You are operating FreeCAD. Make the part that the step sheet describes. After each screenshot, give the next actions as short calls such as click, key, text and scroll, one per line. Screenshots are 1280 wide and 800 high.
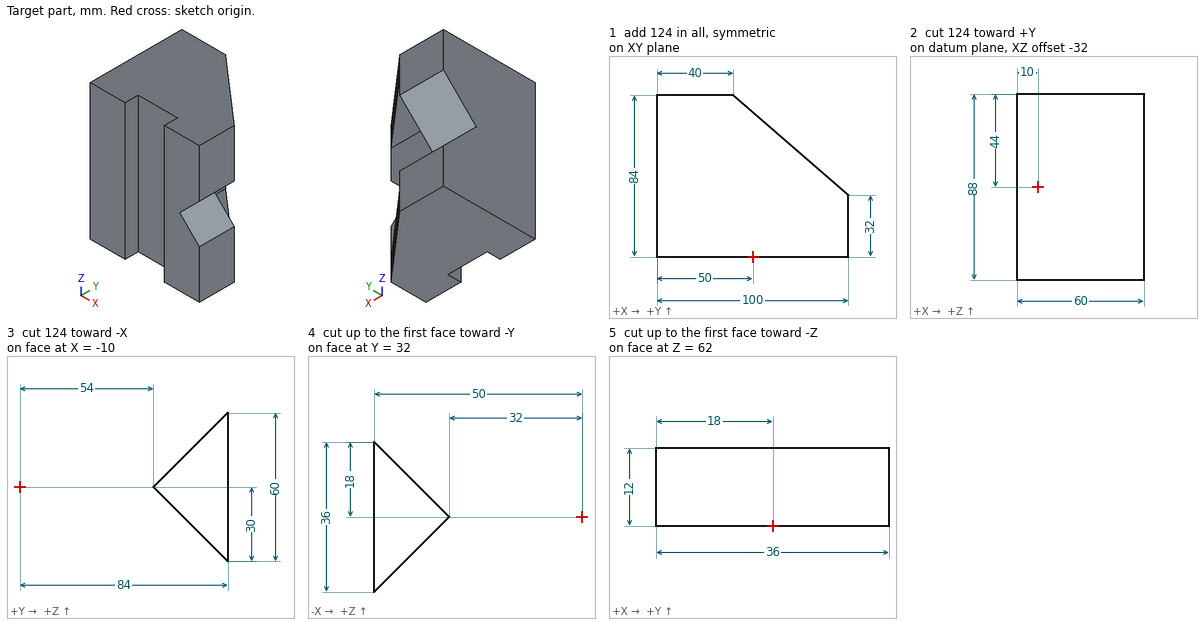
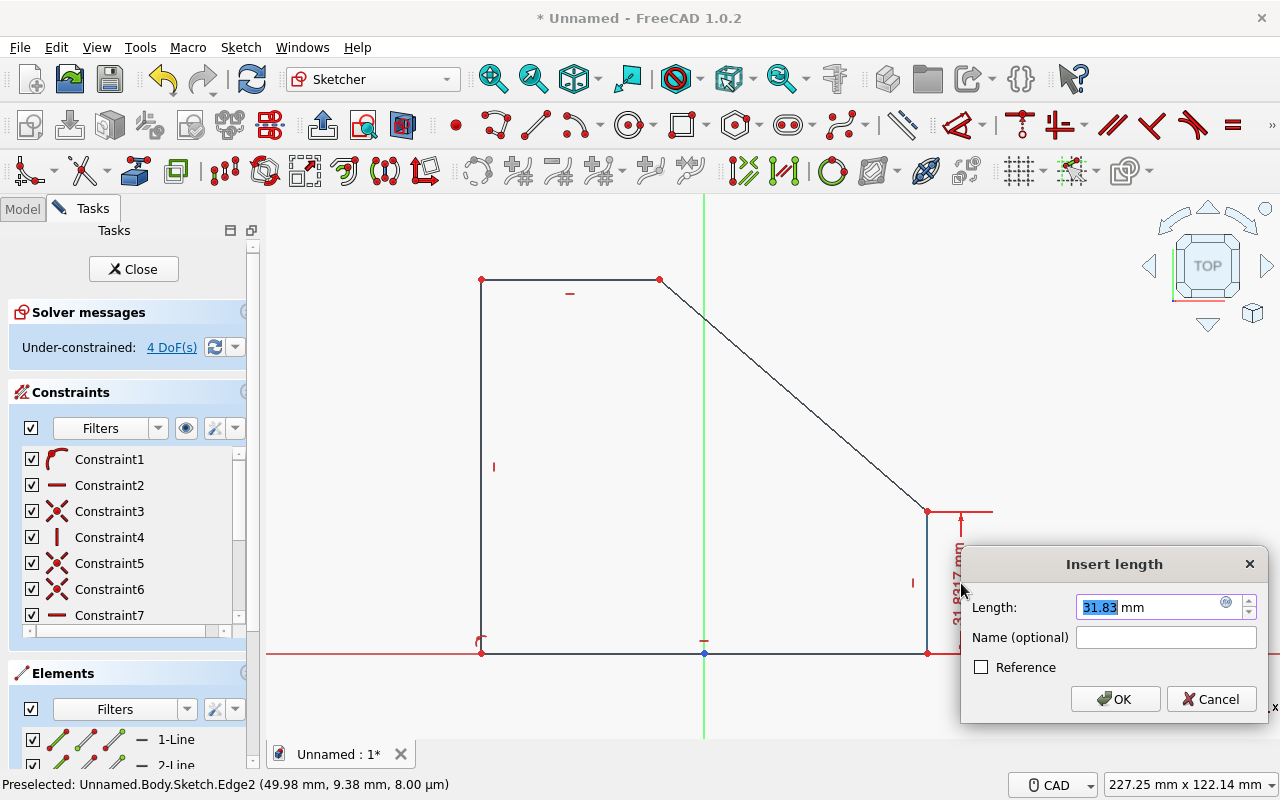
text(32)
key(Return)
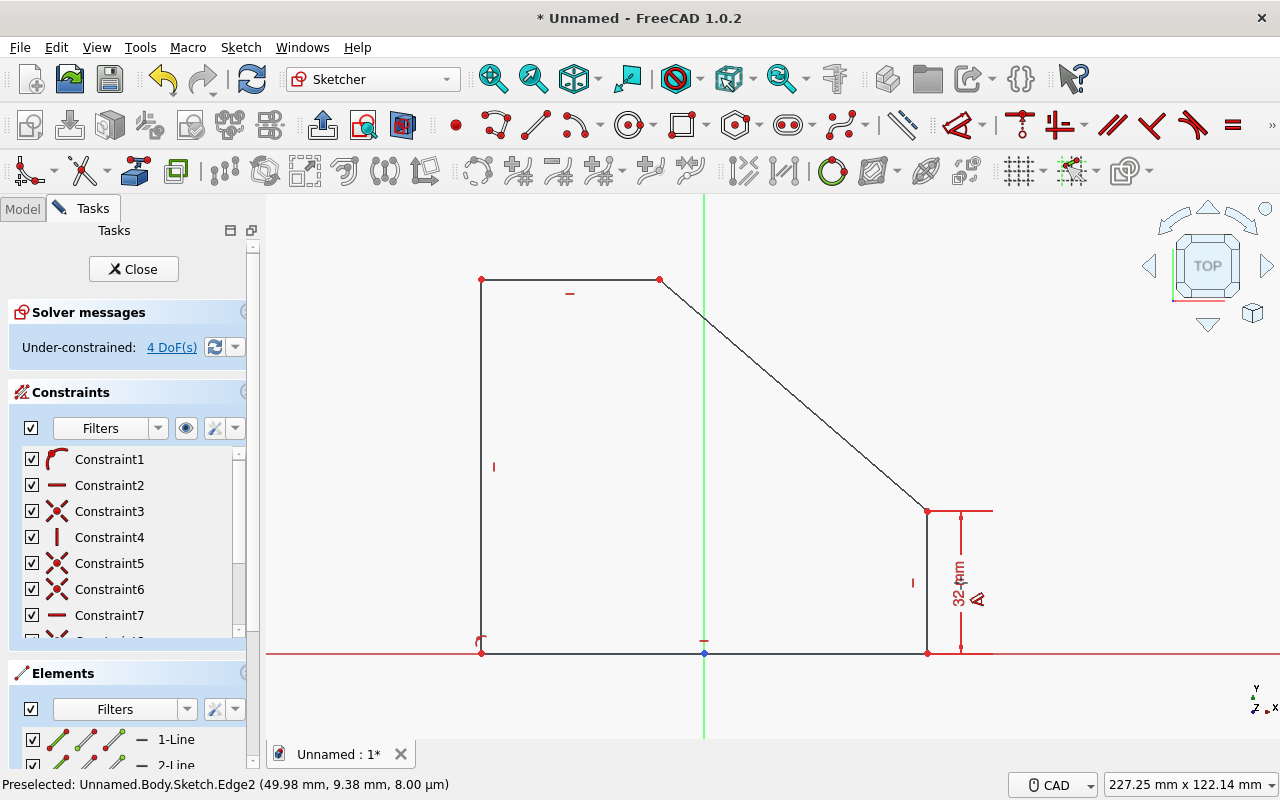
click(606, 280)
click(570, 246)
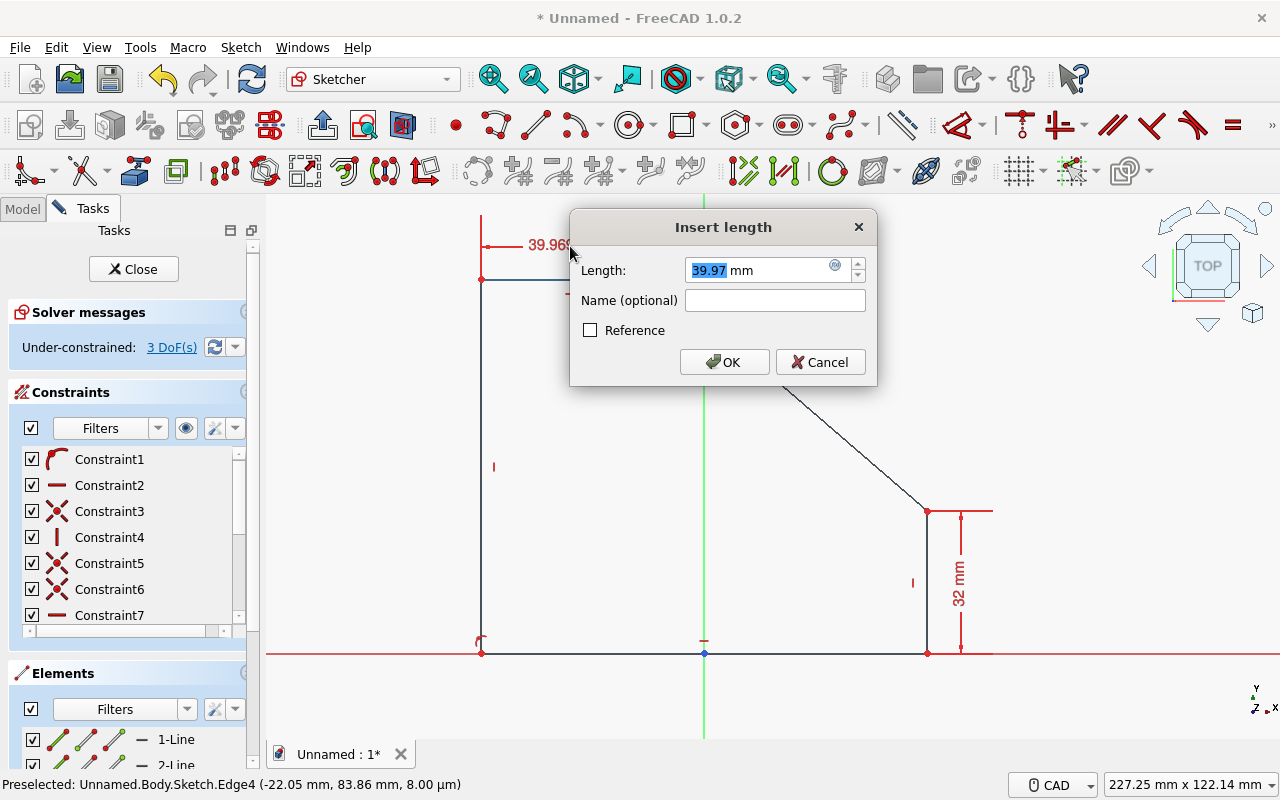
text(40)
key(Return)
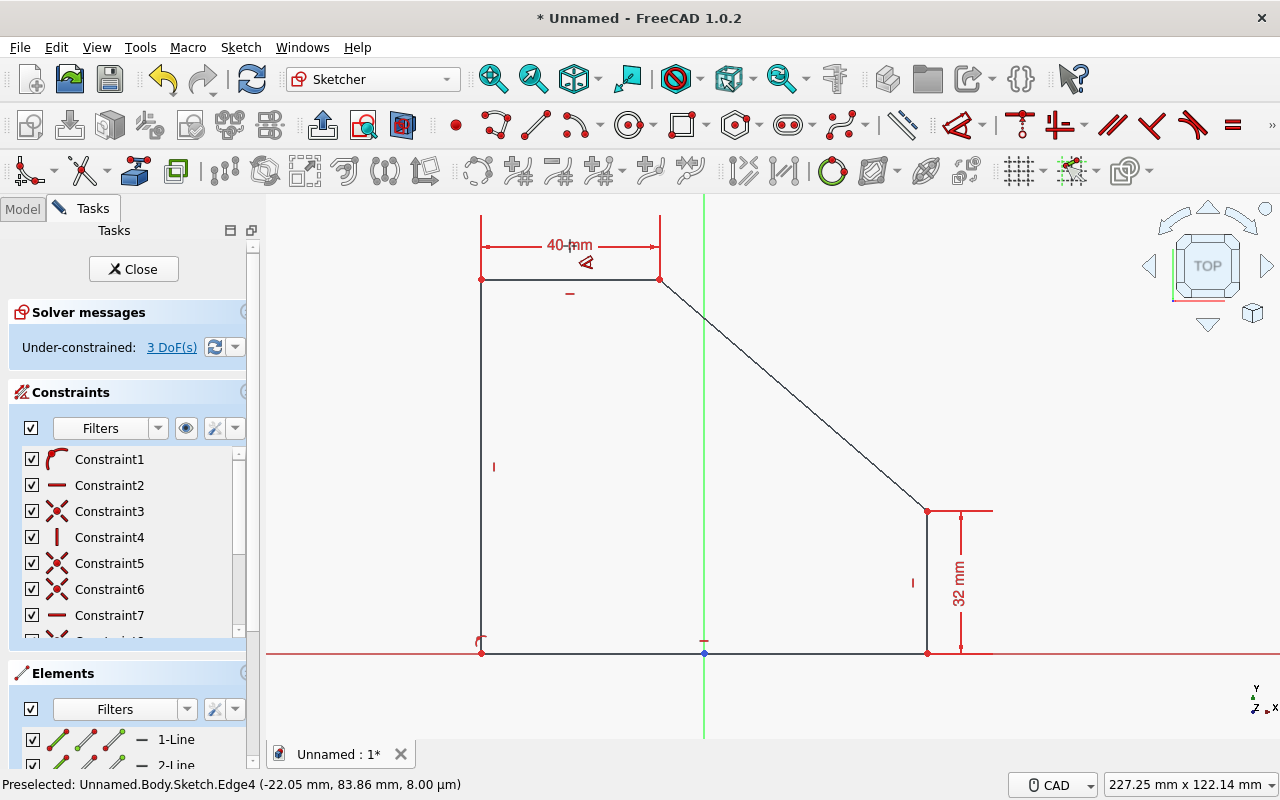
click(481, 392)
click(447, 467)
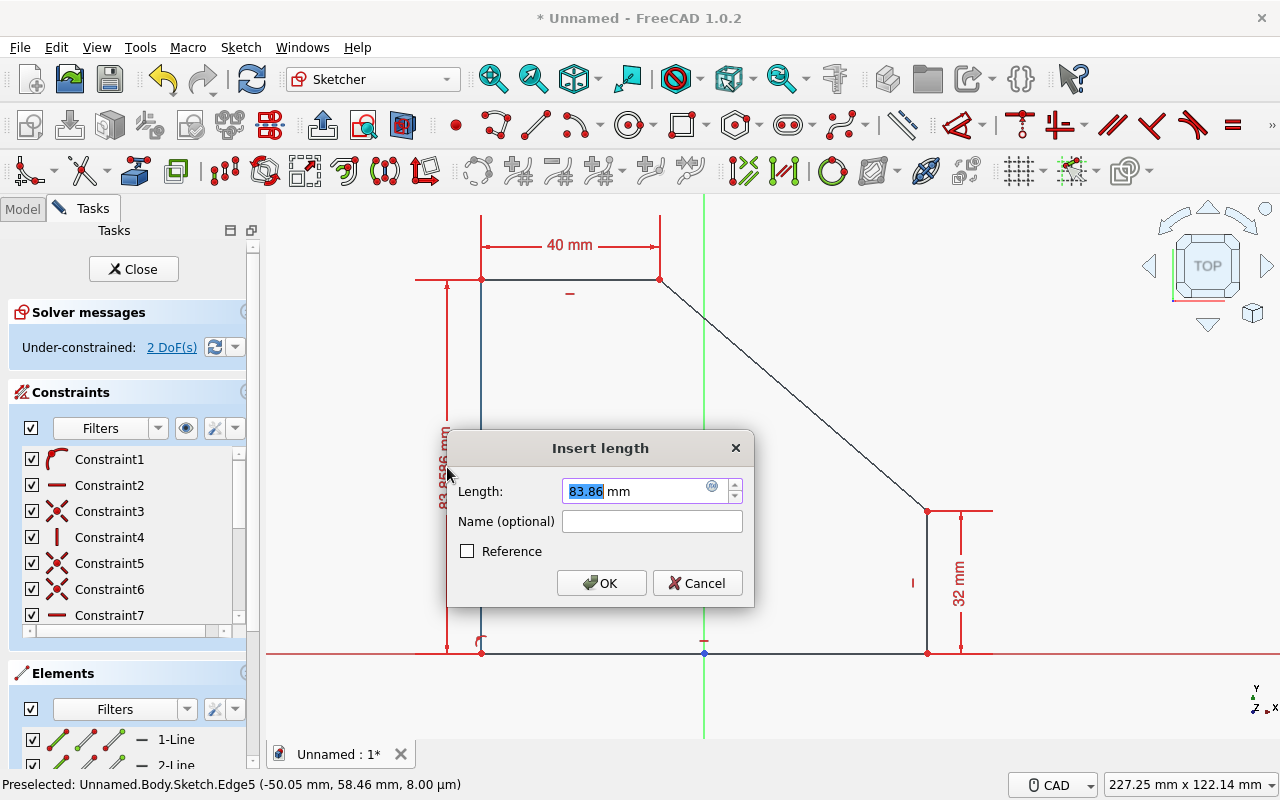
text(84)
key(Return)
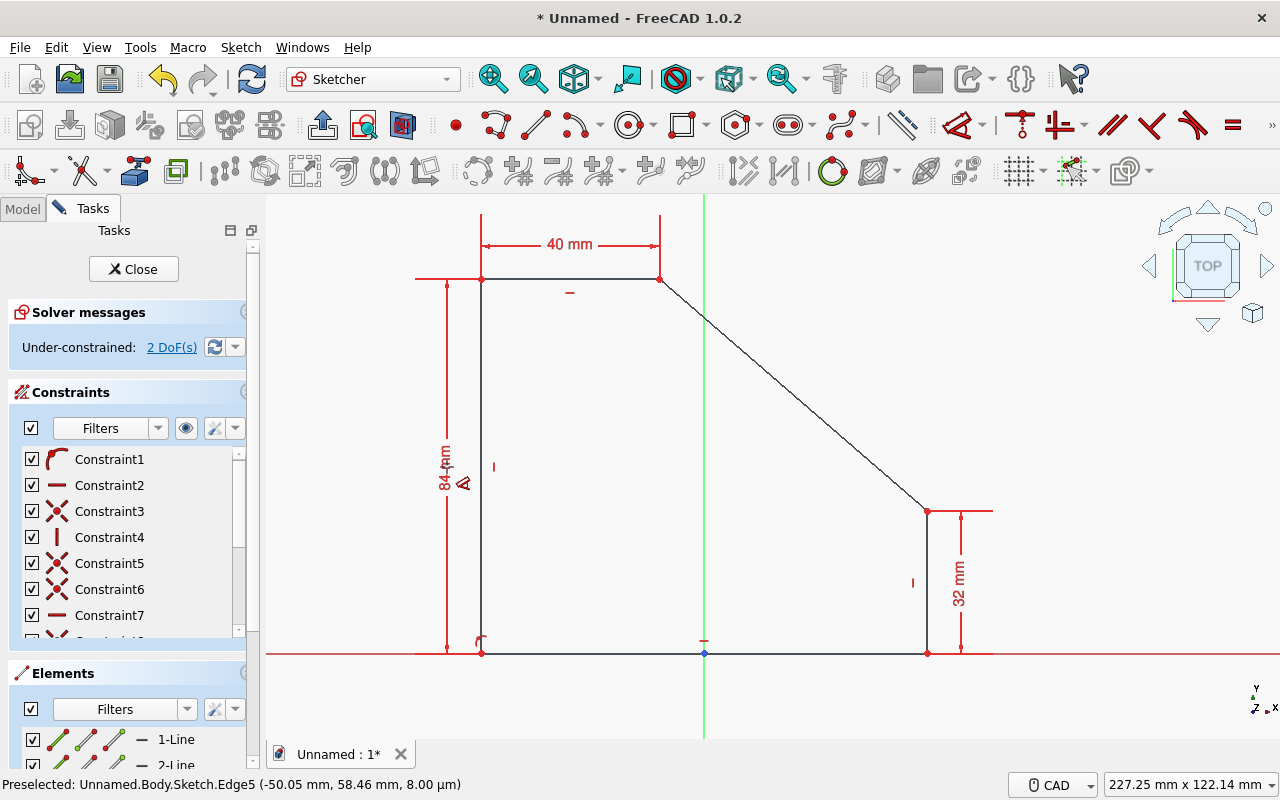
click(615, 654)
click(602, 688)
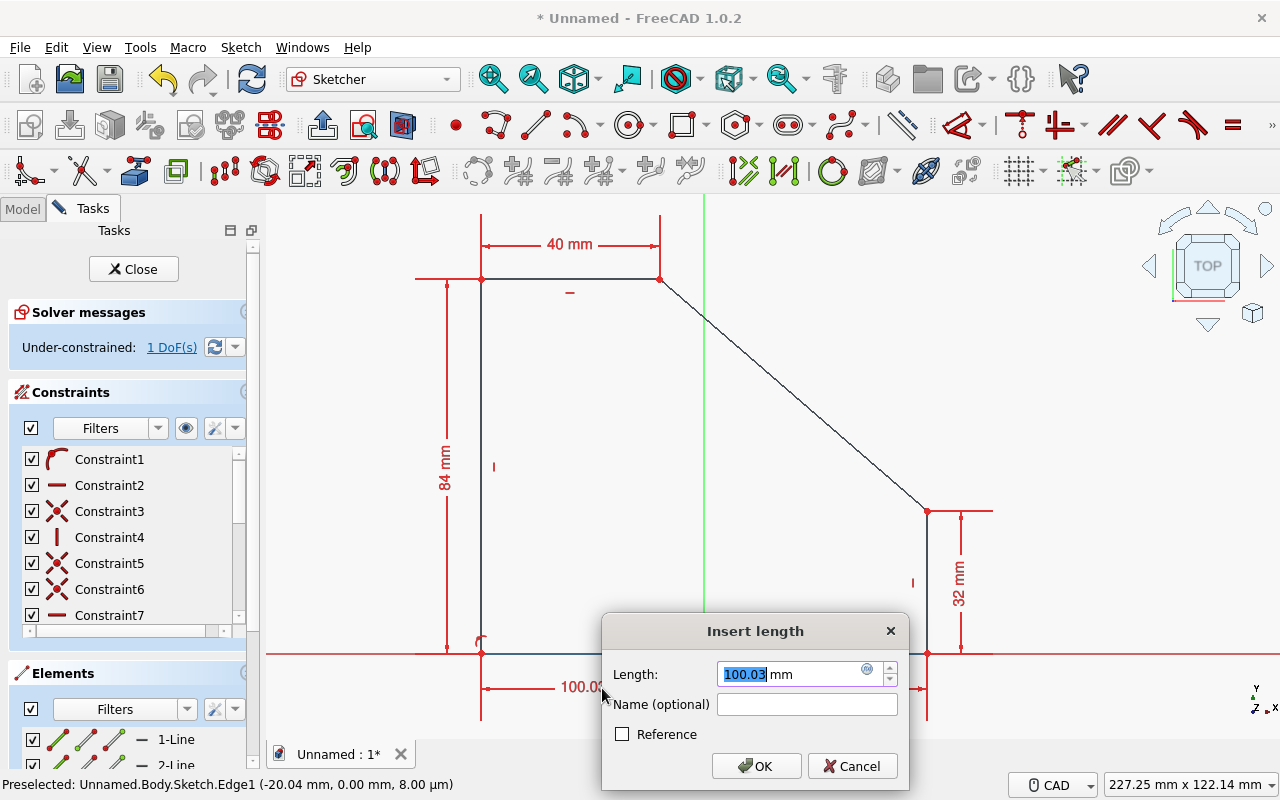
text(100)
key(Return)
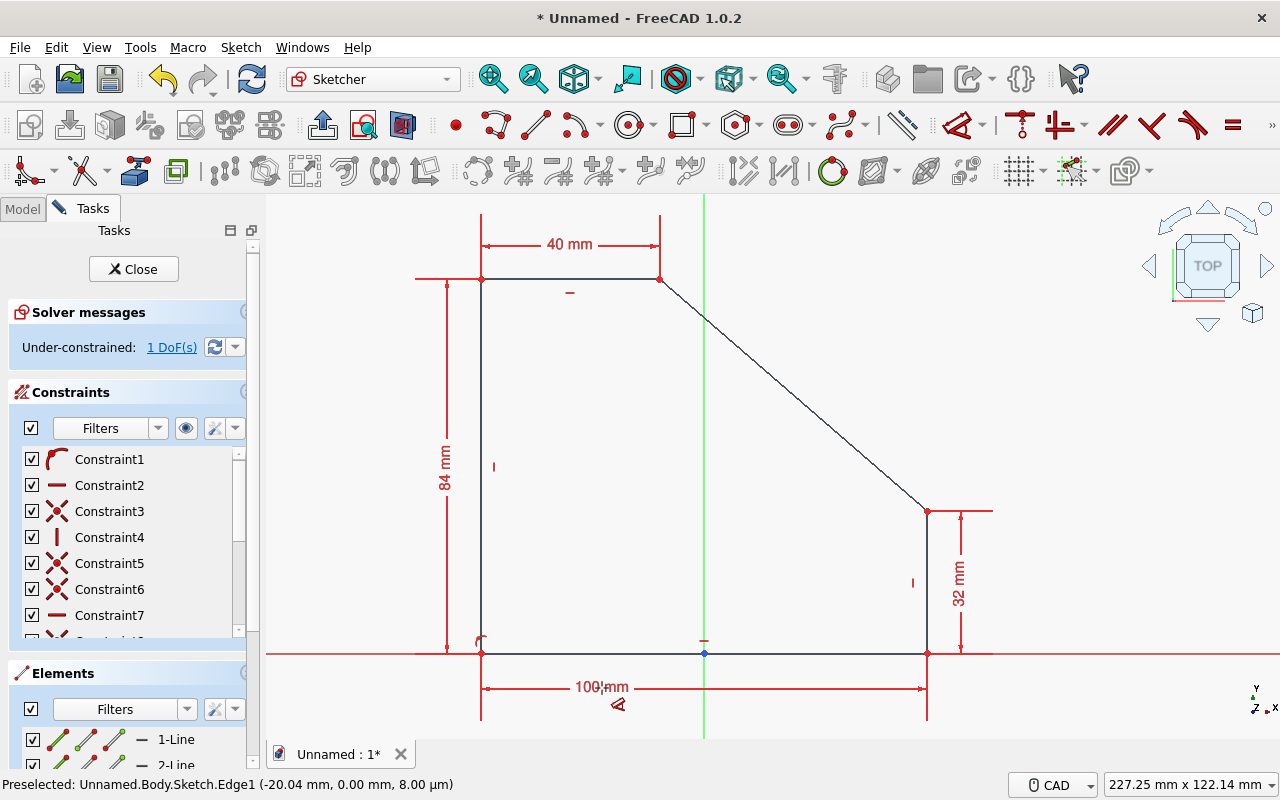
click(481, 654)
click(515, 688)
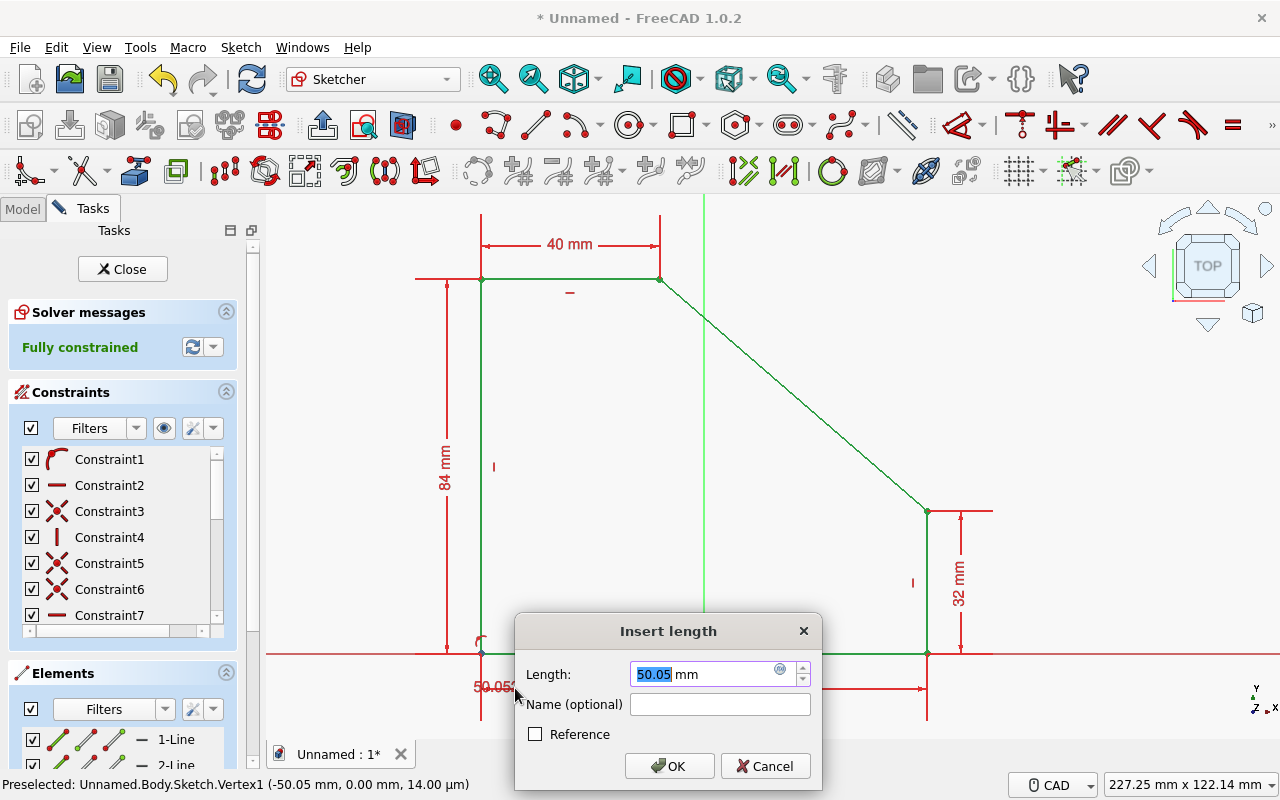
text(50)
key(Return)
key(Escape)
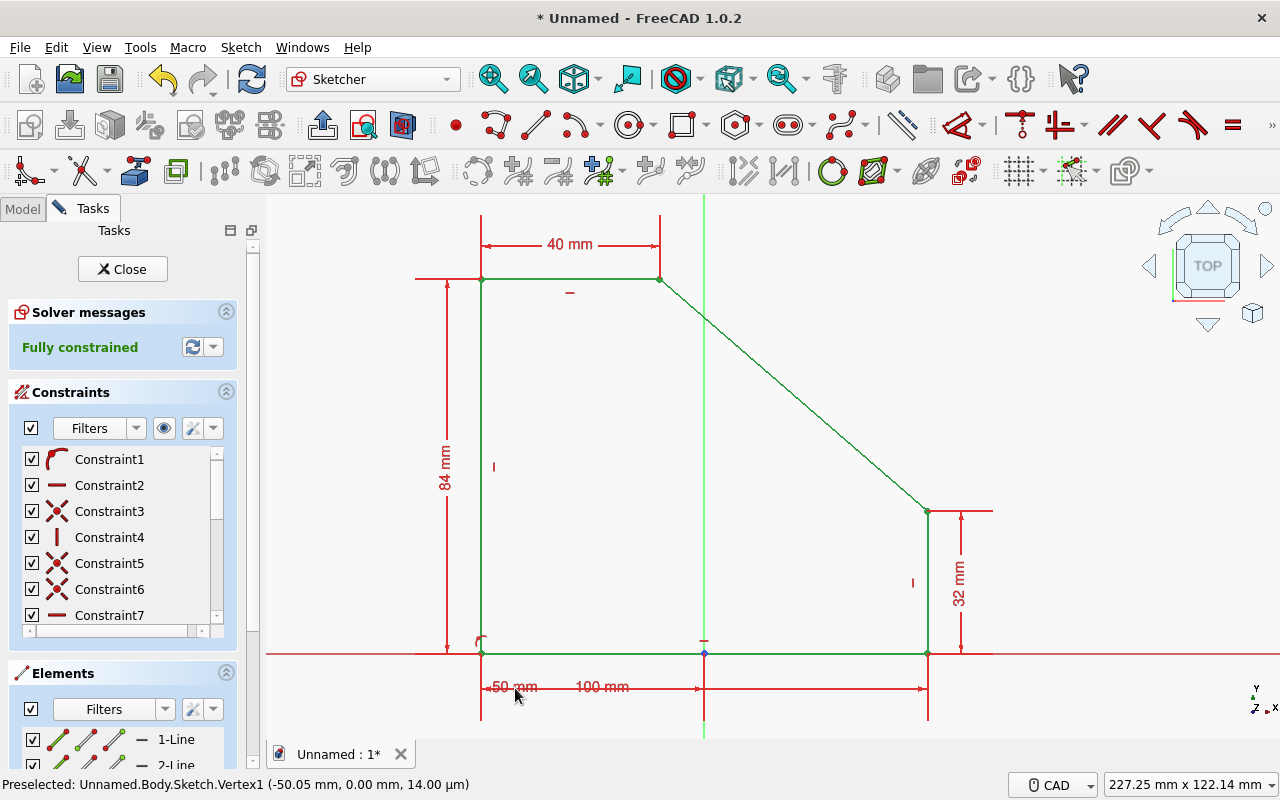
click(123, 269)